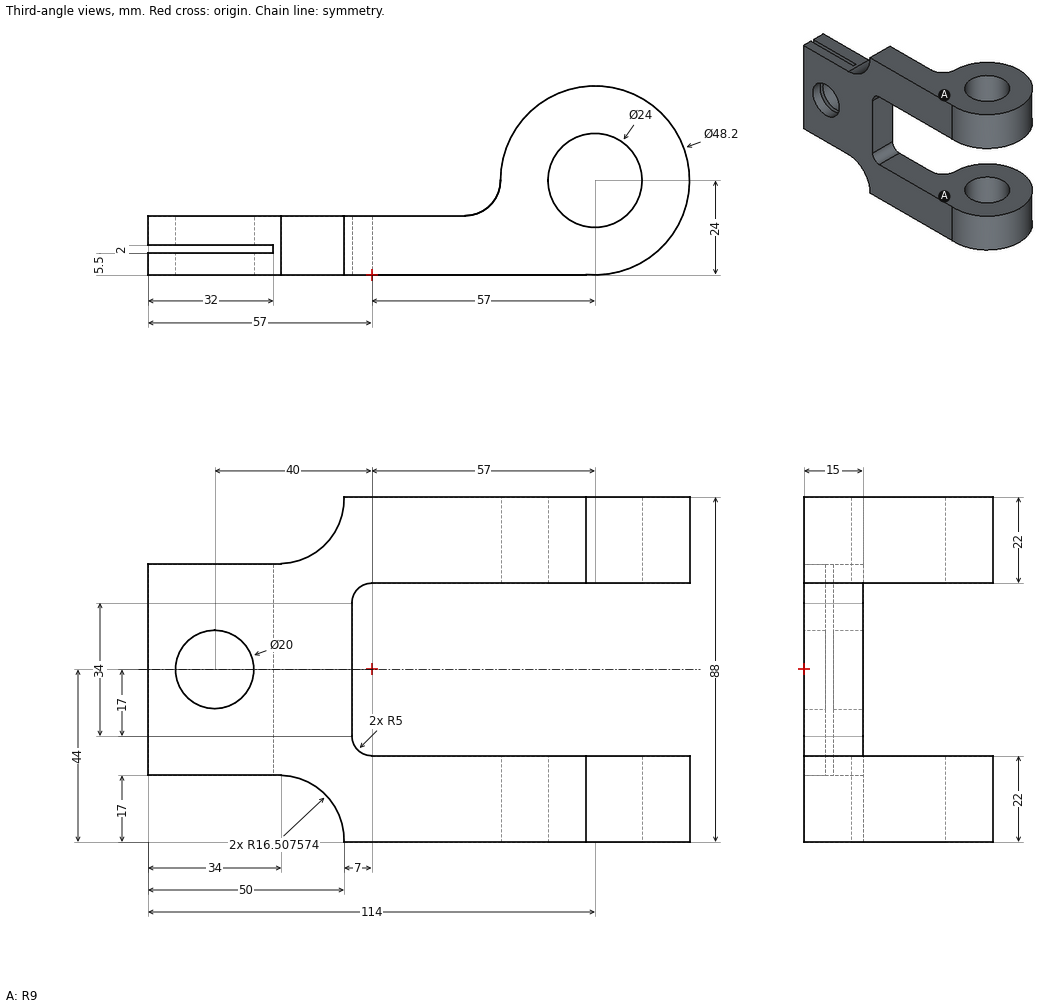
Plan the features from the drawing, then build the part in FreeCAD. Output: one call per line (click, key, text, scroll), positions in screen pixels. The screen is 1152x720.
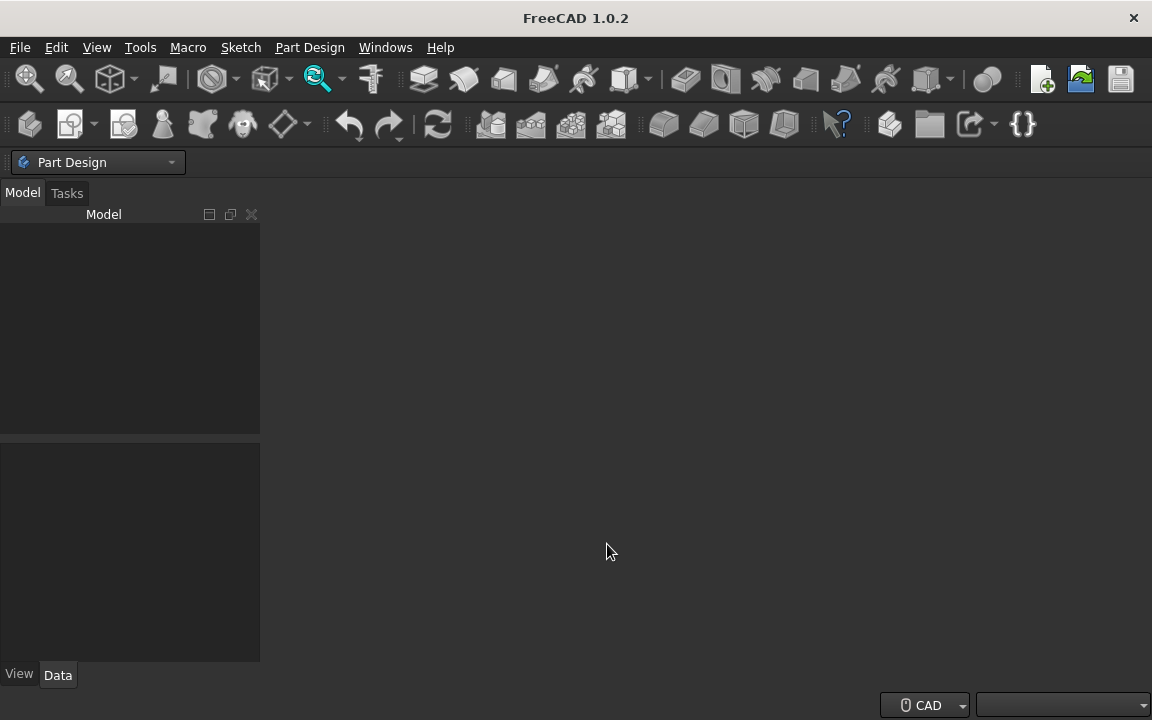
key(ctrl+n)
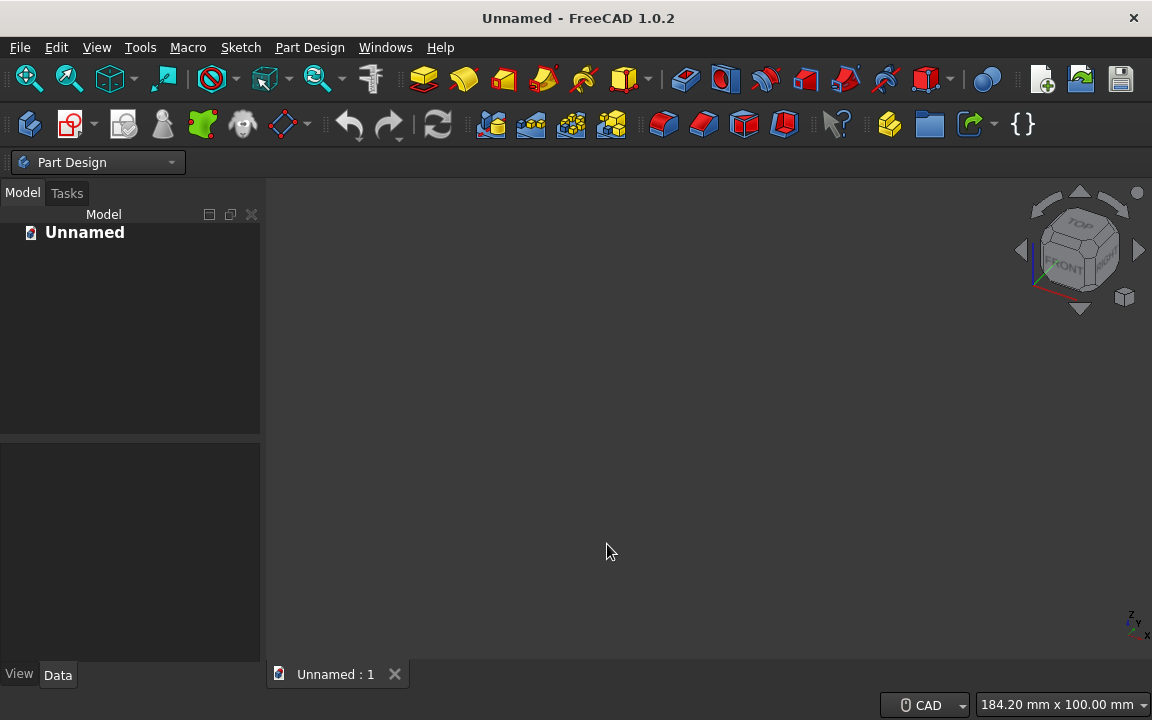
click(70, 124)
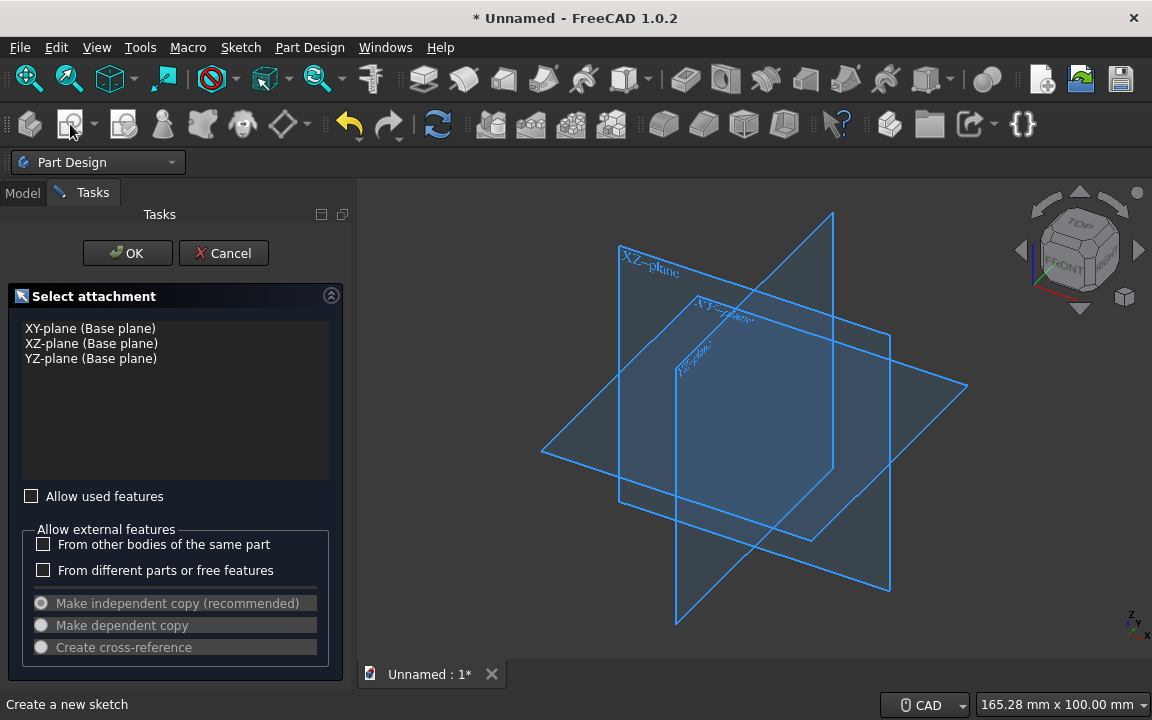
click(82, 344)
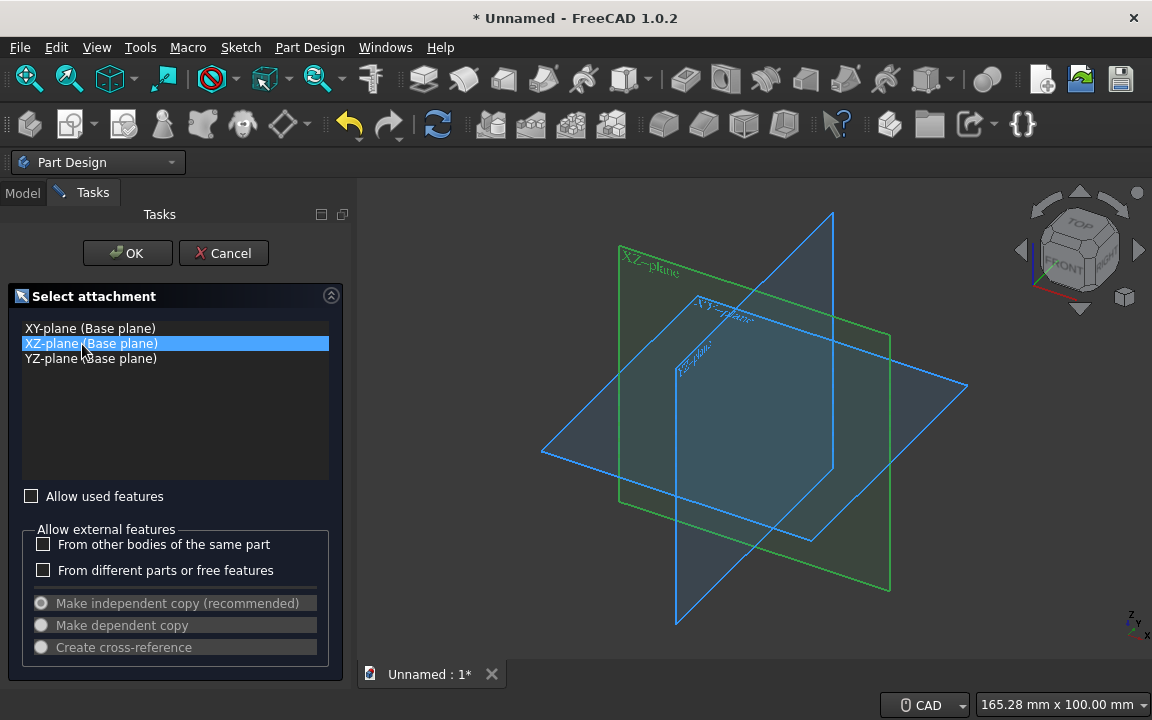
click(128, 253)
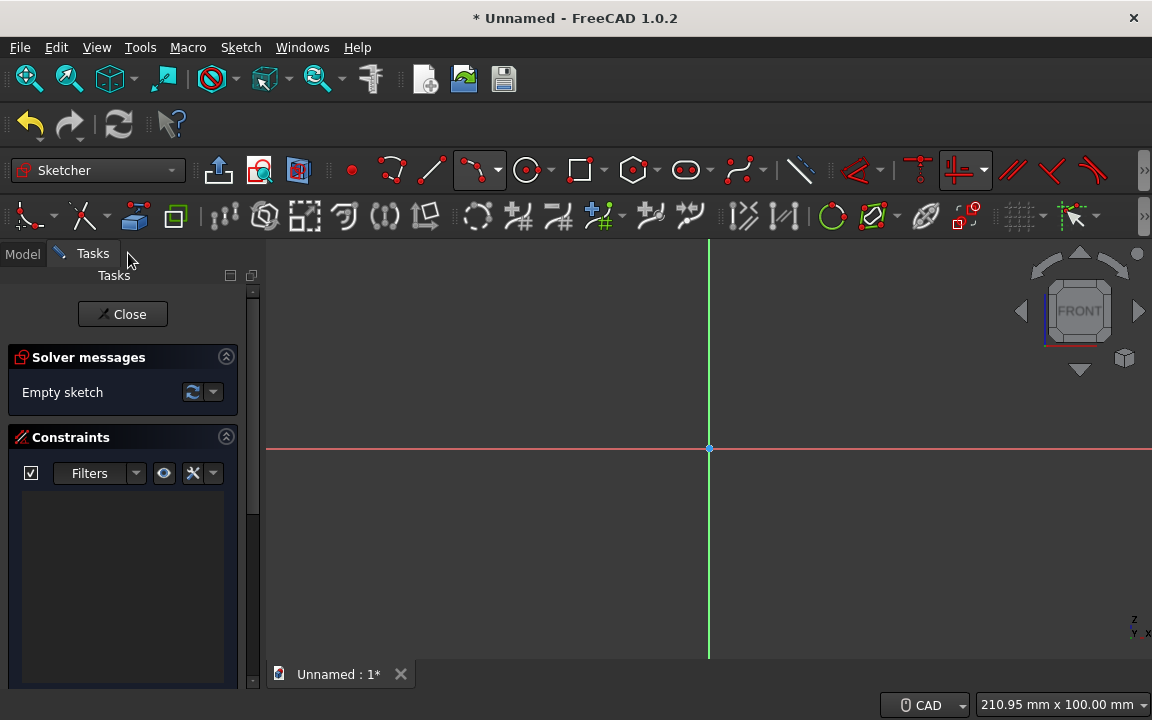
scroll(501, 449, down, 2)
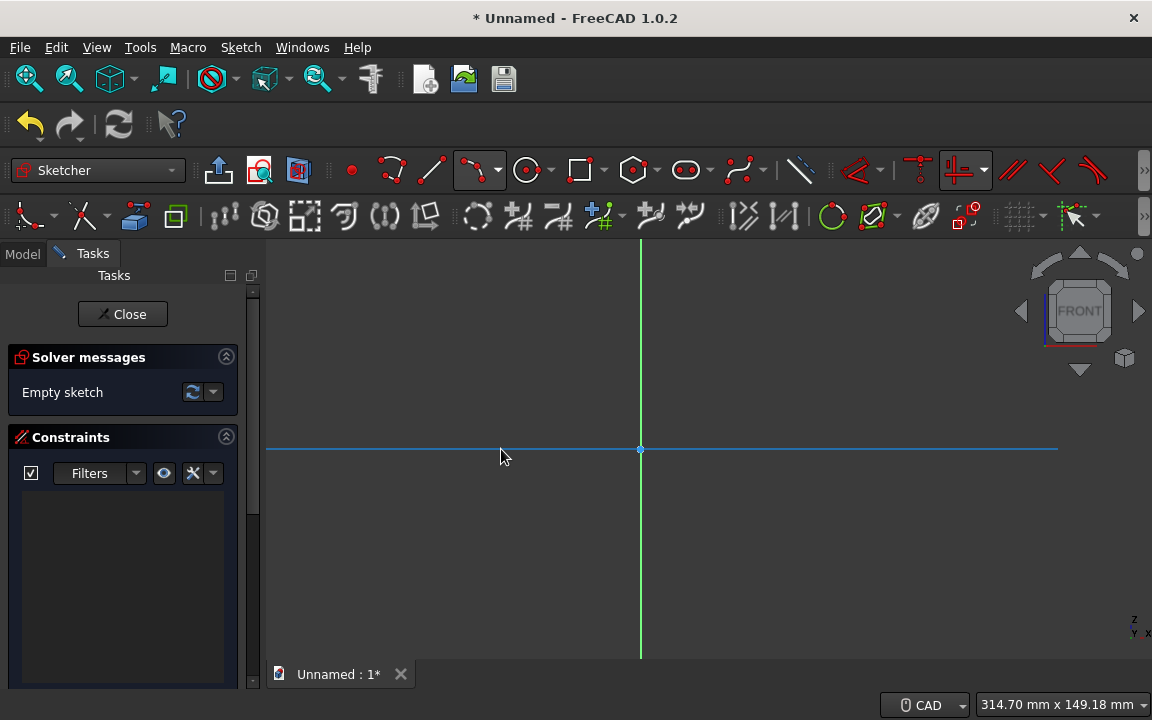
key(g)
key(v)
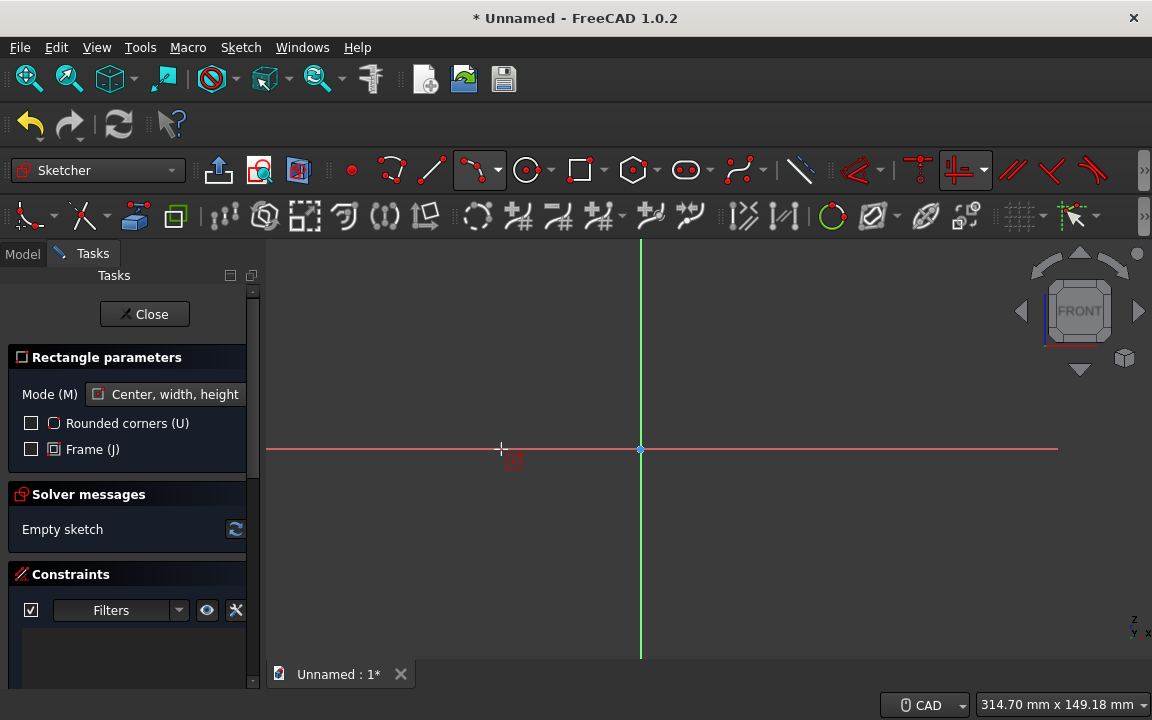
click(641, 449)
move(801, 325)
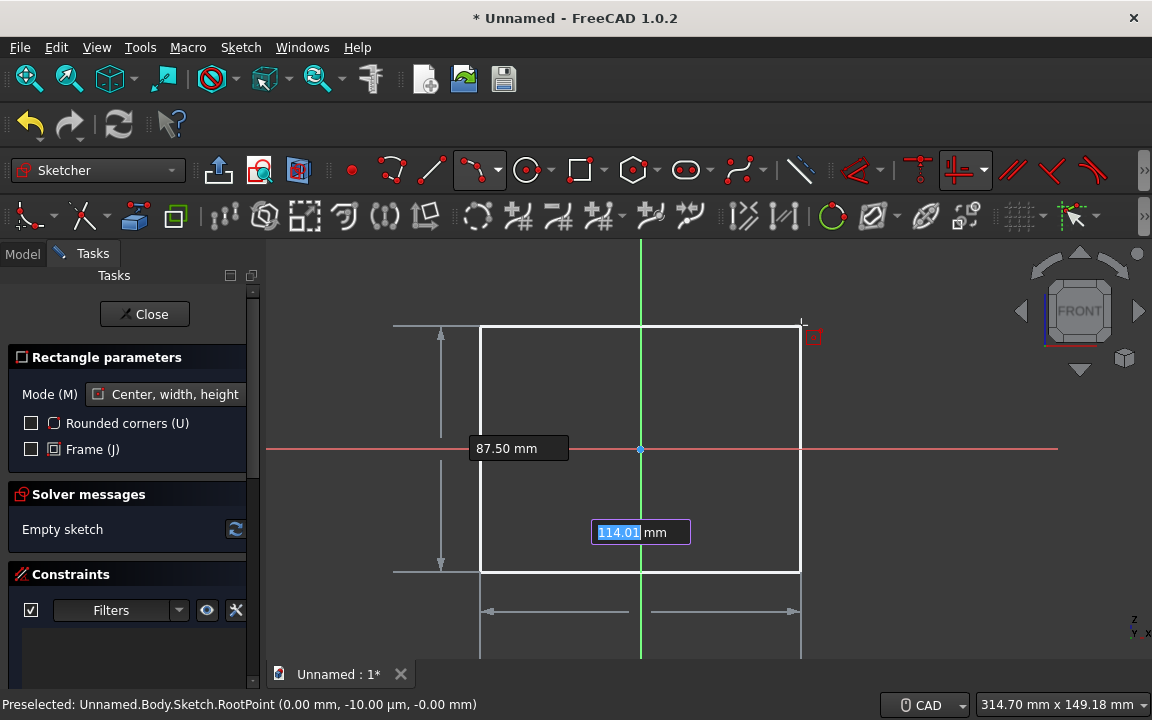
text(114)
key(Tab)
text(88)
key(Return)
key(Escape)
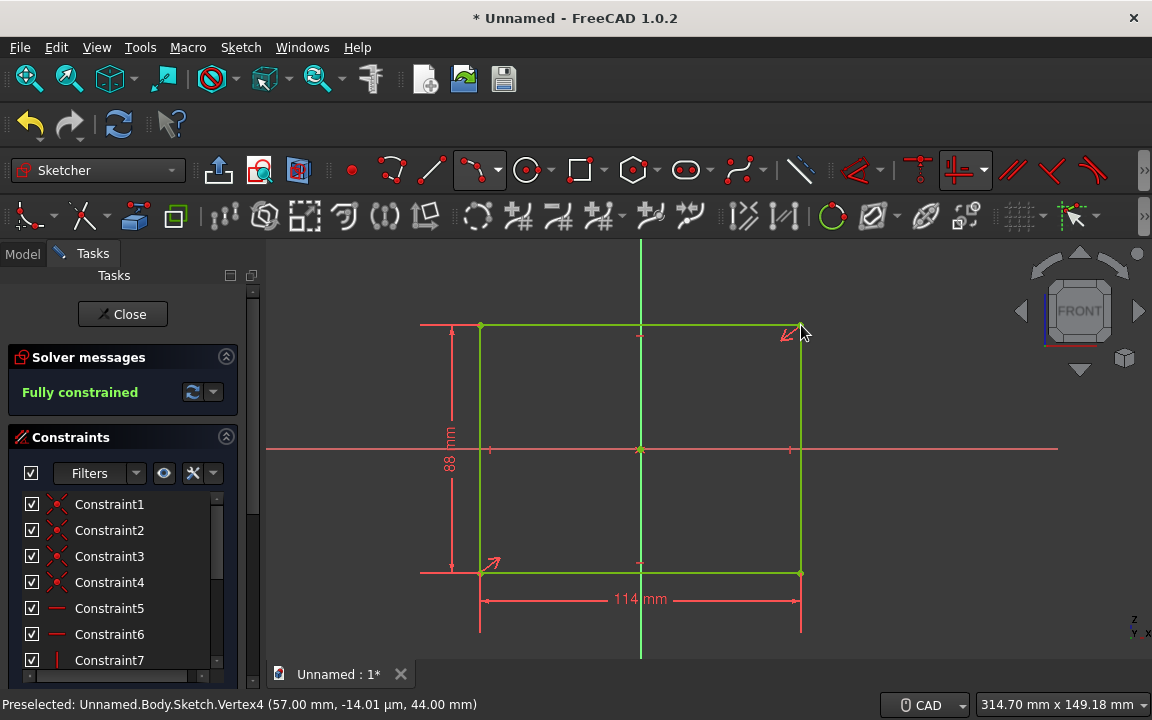
click(123, 314)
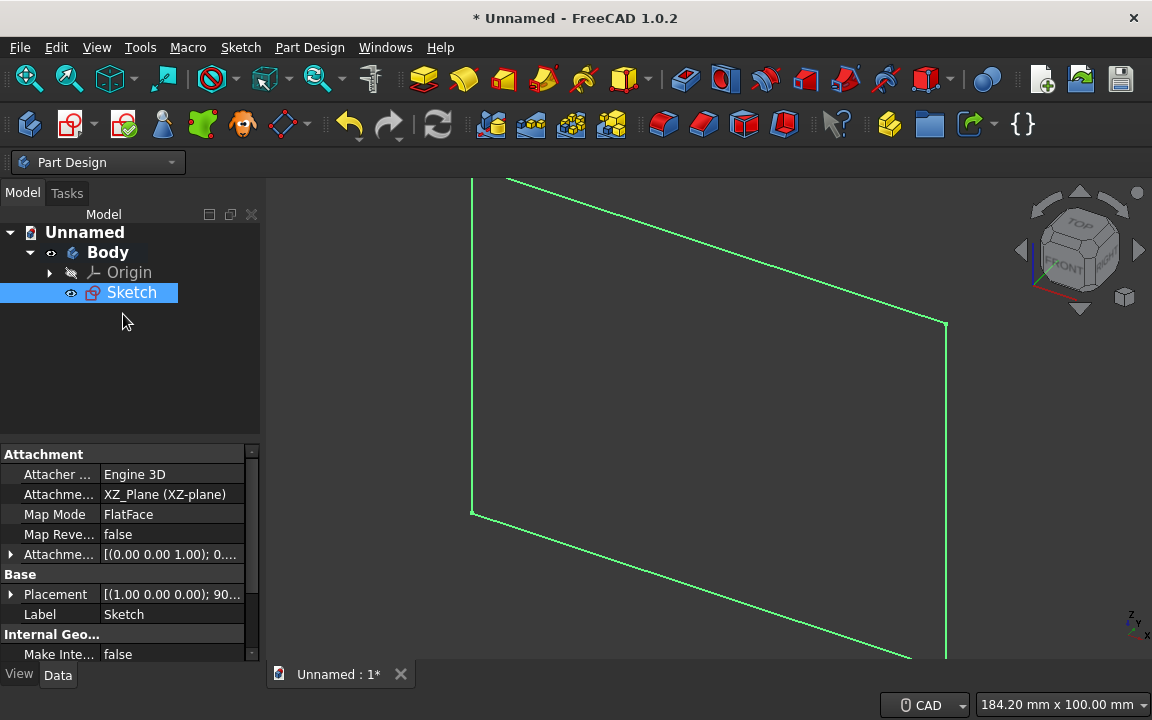
click(424, 80)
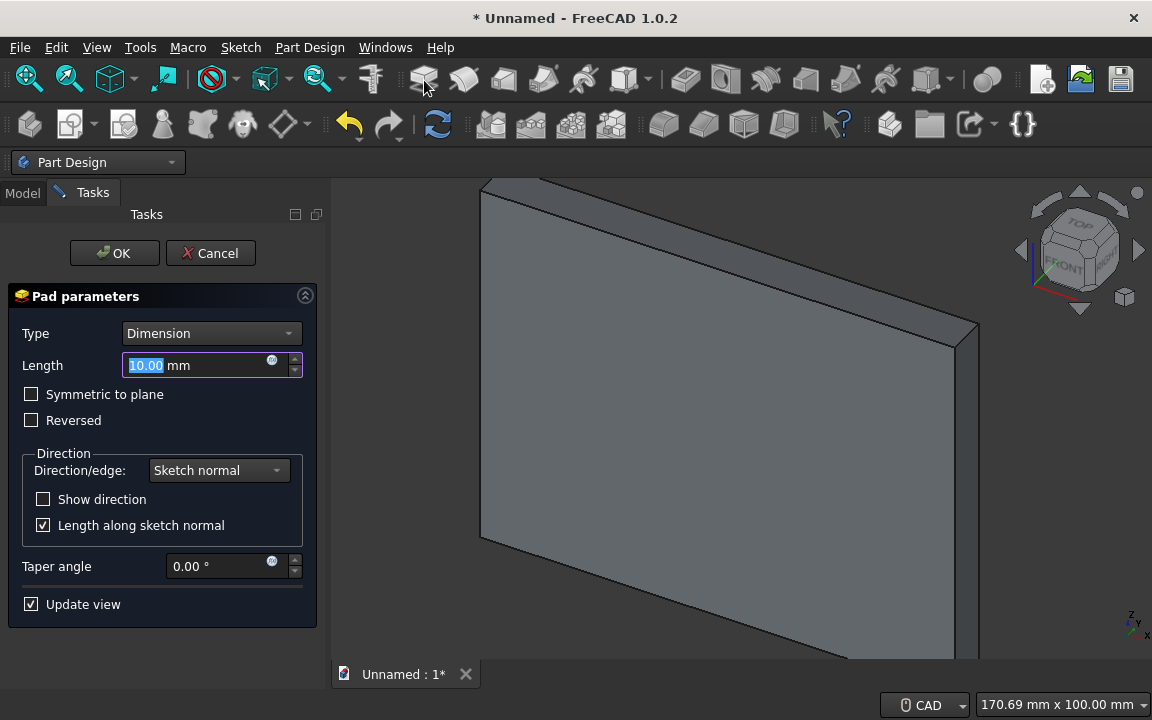
text(15)
key(Tab)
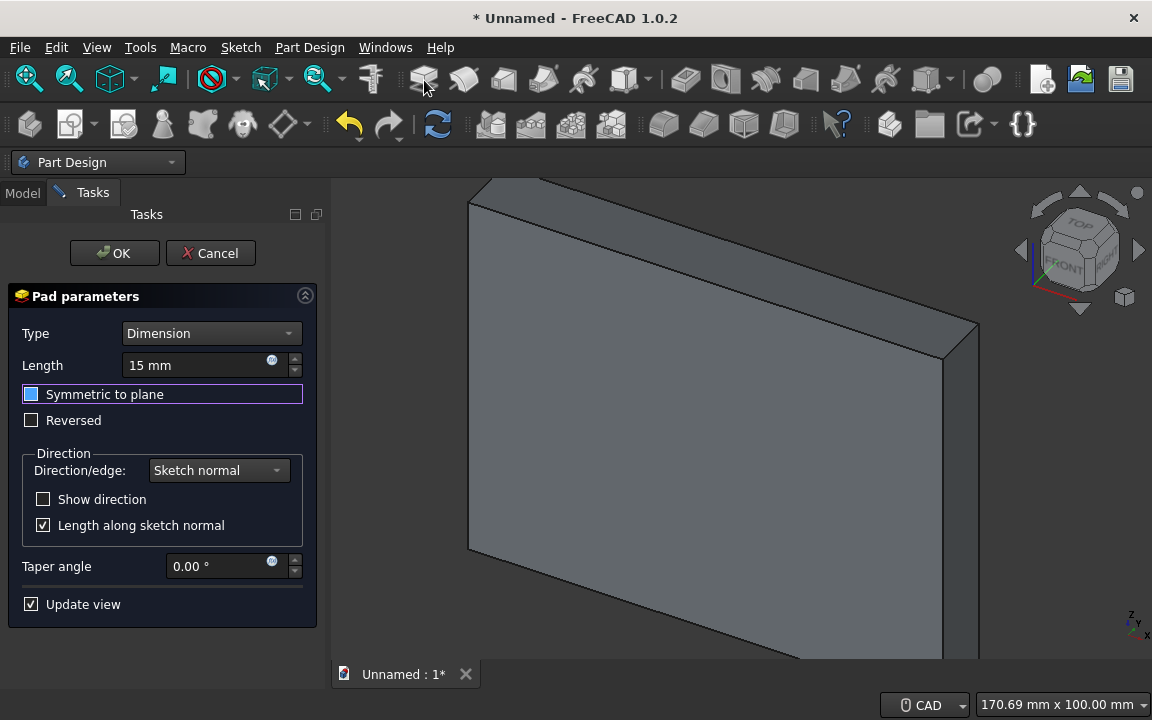
click(30, 420)